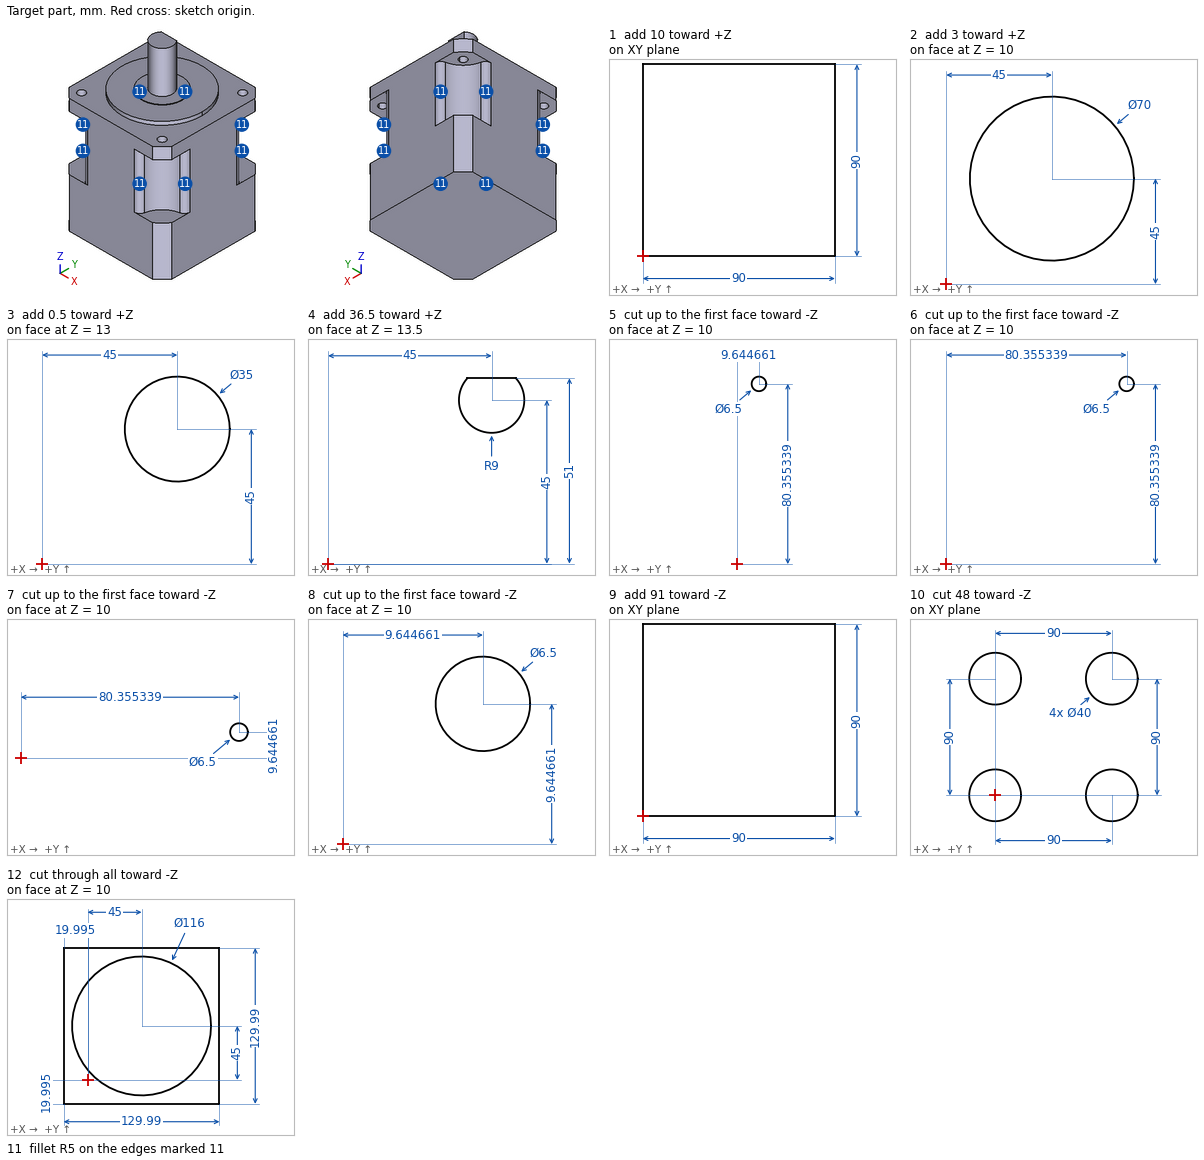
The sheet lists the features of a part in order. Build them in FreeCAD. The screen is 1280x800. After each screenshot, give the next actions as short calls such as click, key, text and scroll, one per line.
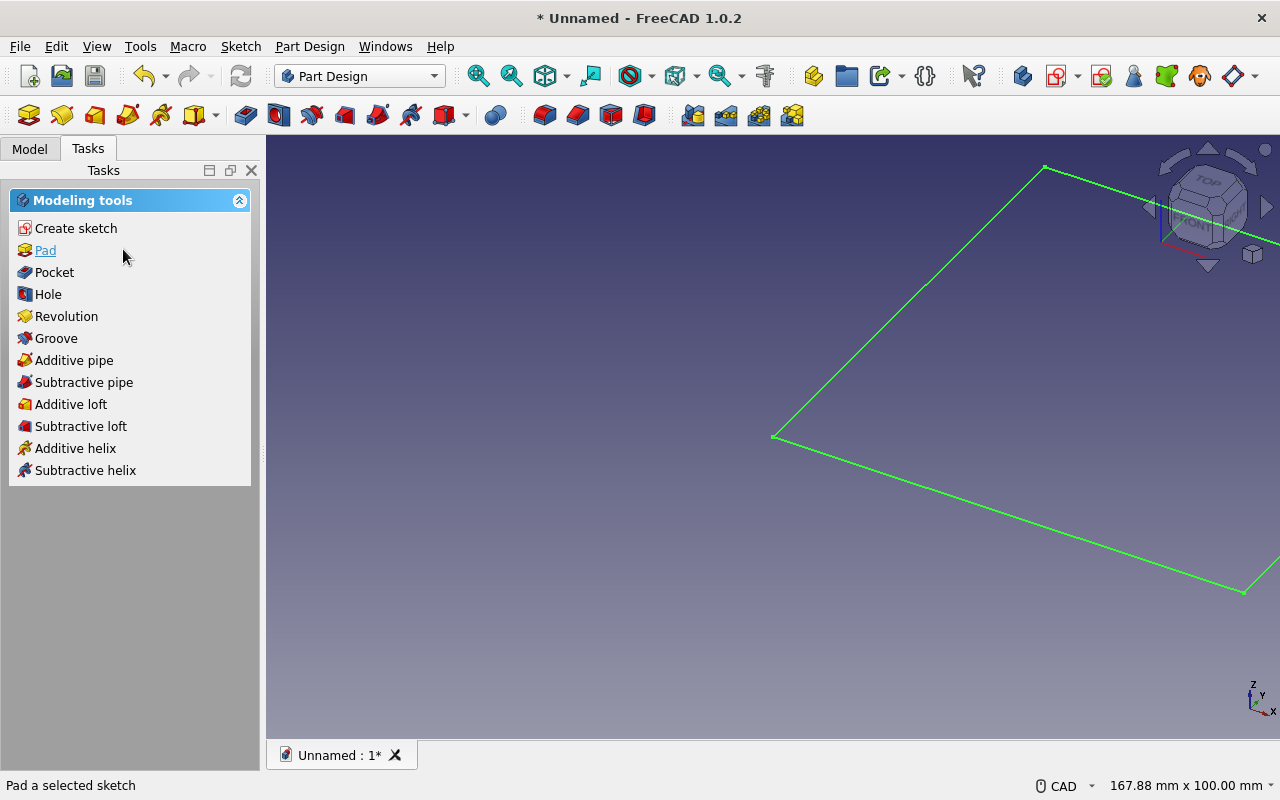
click(29, 116)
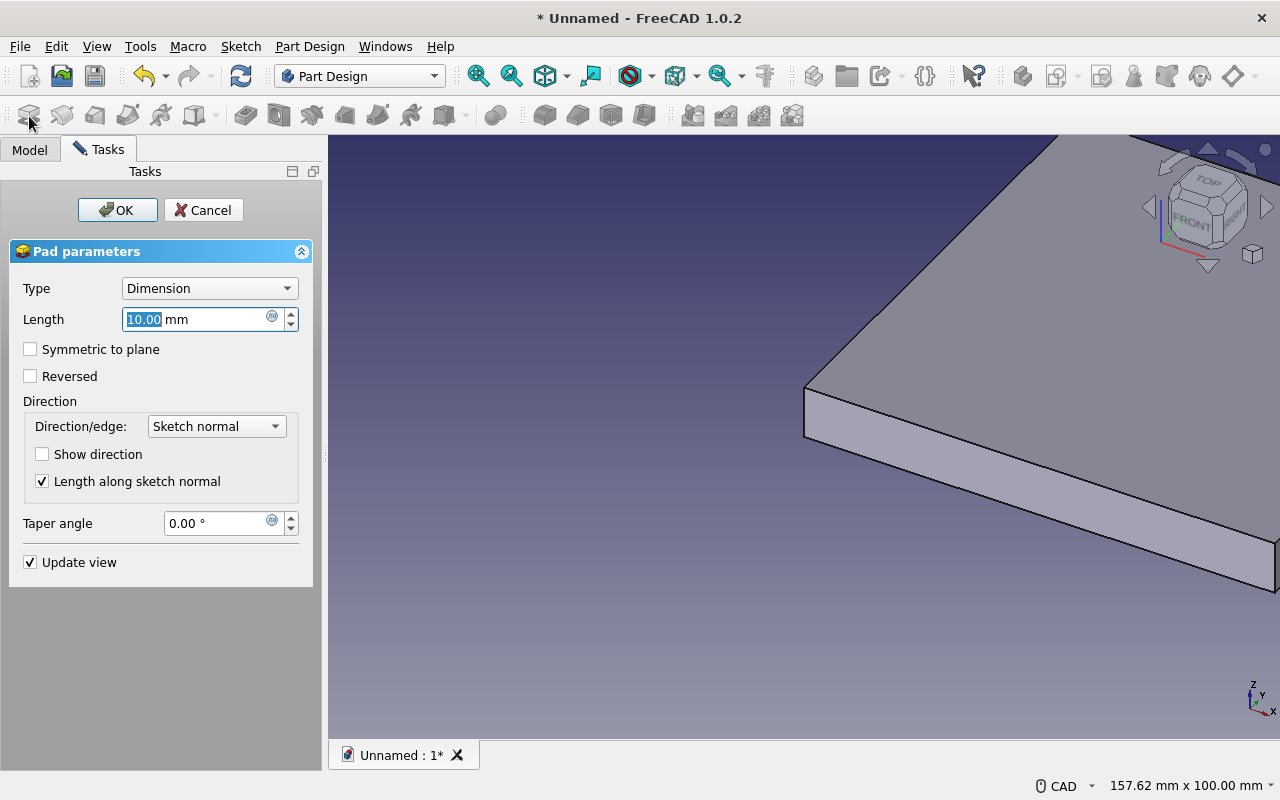
text(10)
key(Tab)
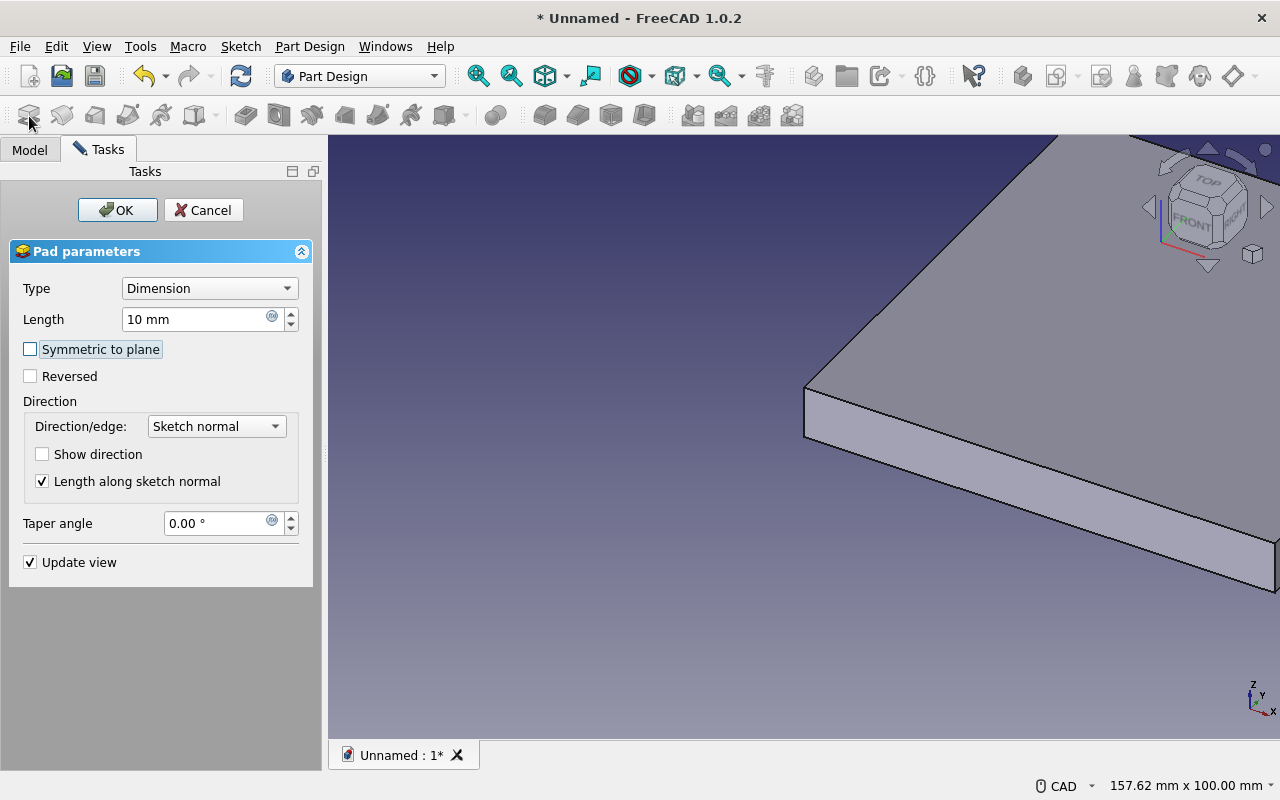
click(118, 210)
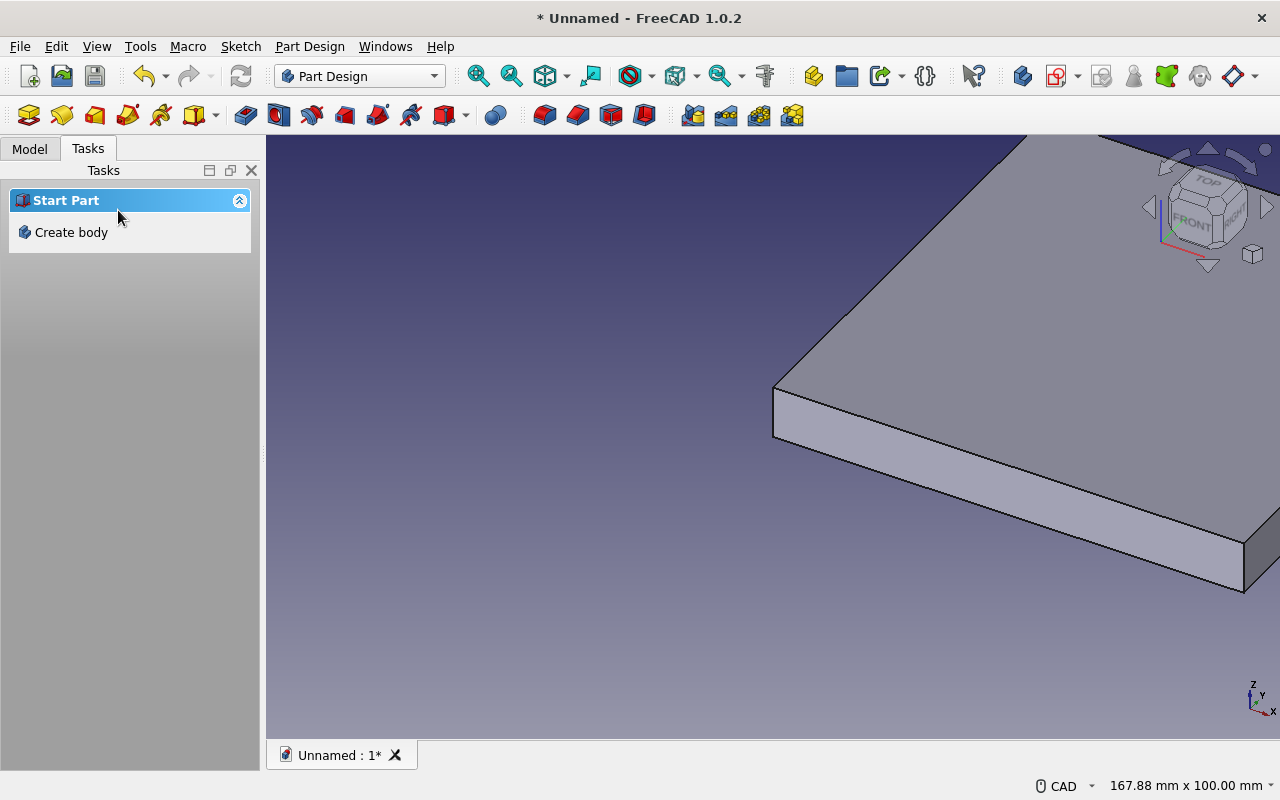
click(479, 76)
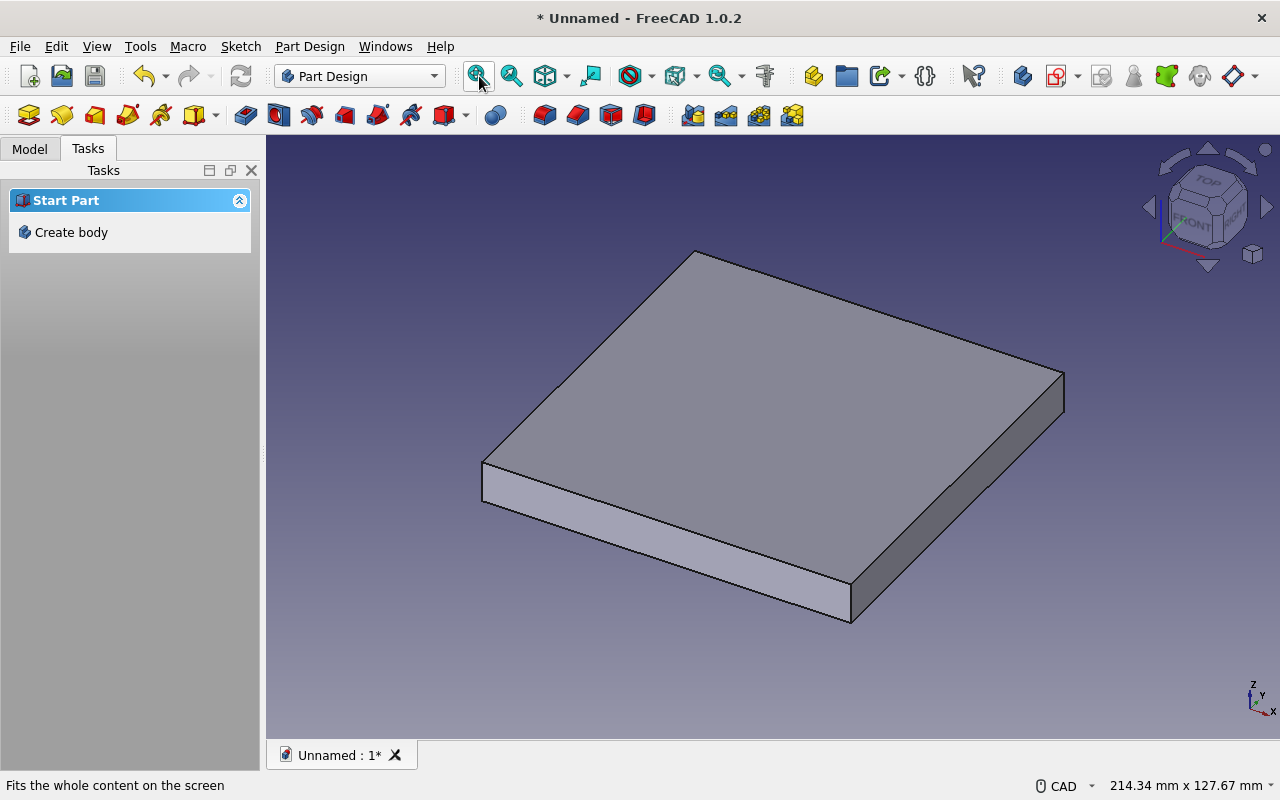
click(773, 417)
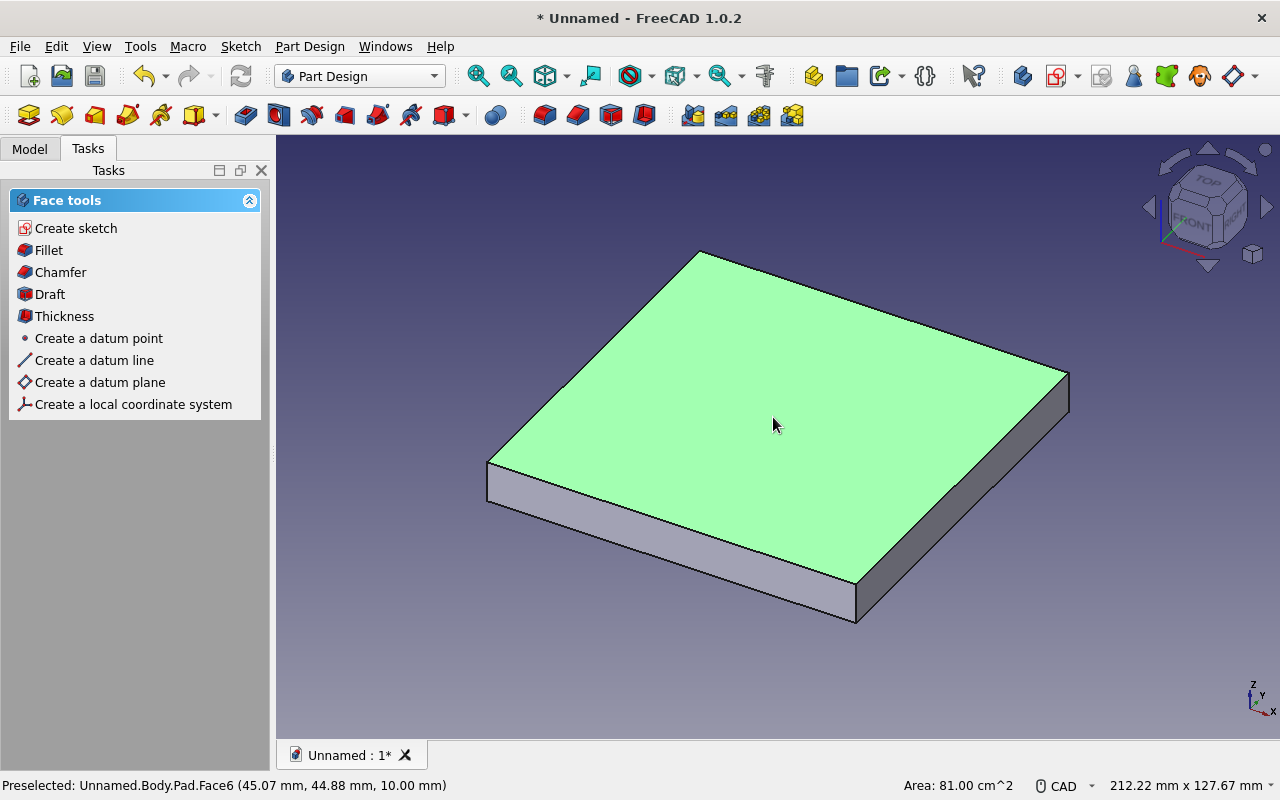
click(1056, 76)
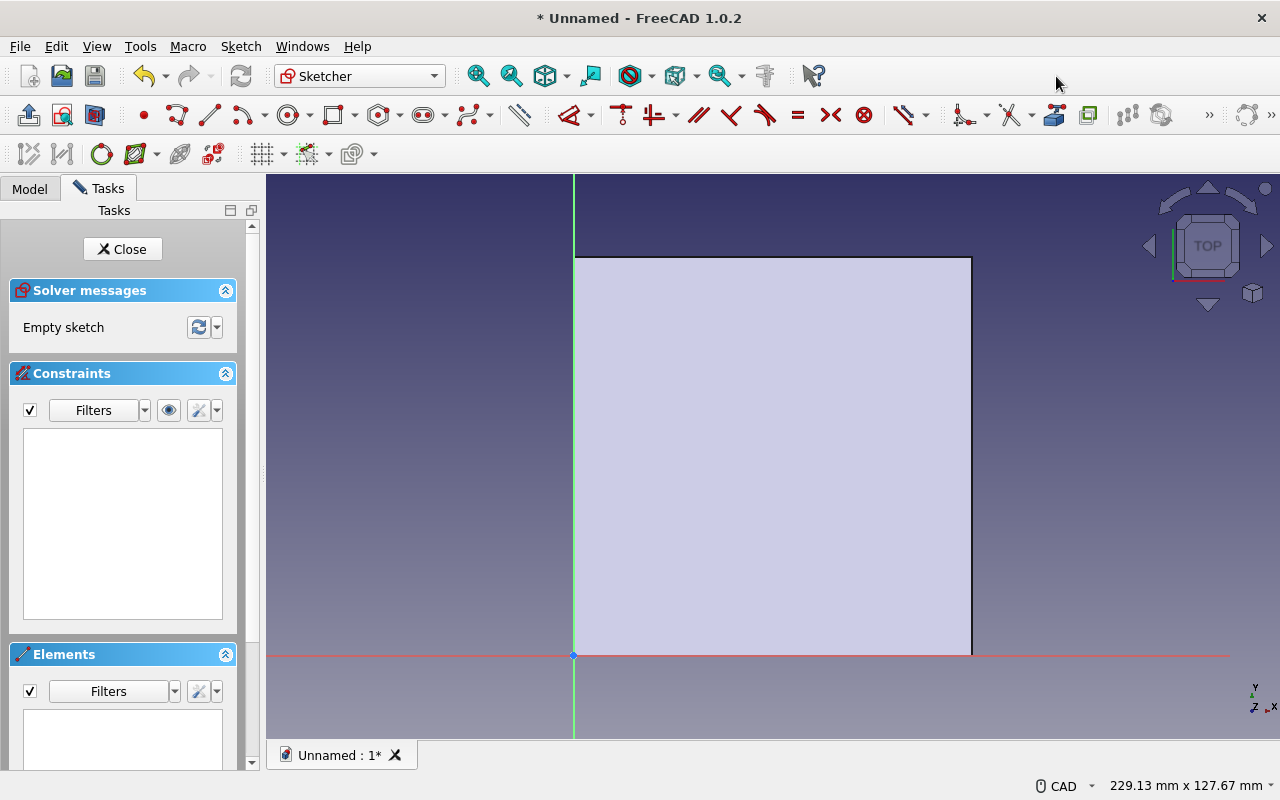
click(288, 116)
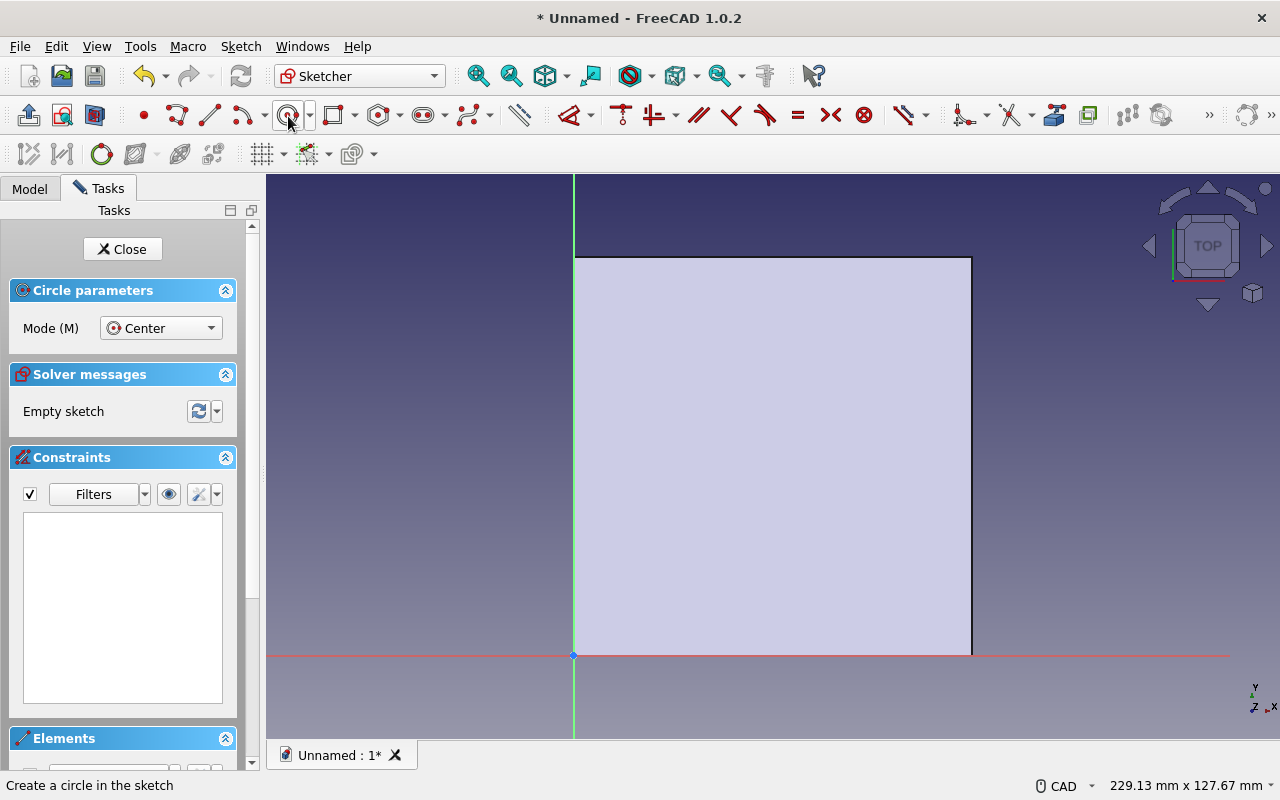
click(773, 456)
move(883, 347)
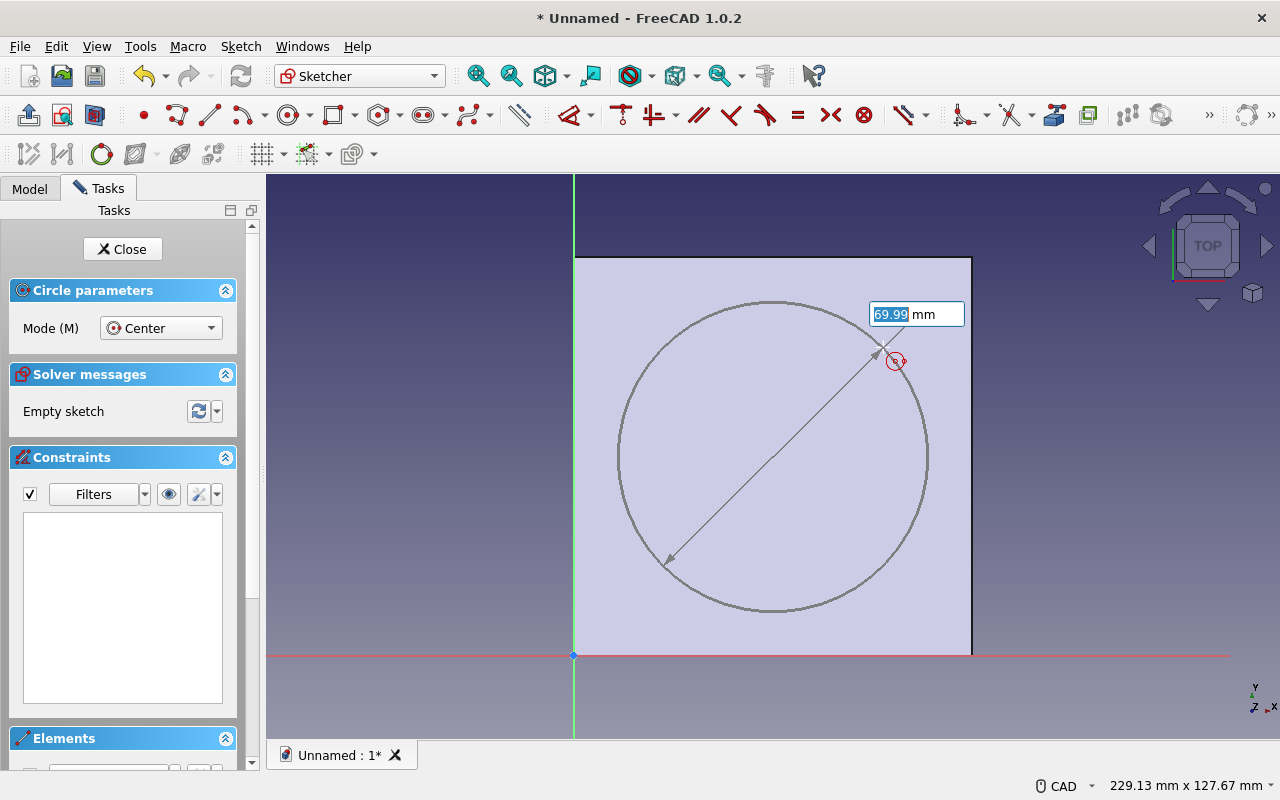
text(70)
key(Return)
key(Escape)